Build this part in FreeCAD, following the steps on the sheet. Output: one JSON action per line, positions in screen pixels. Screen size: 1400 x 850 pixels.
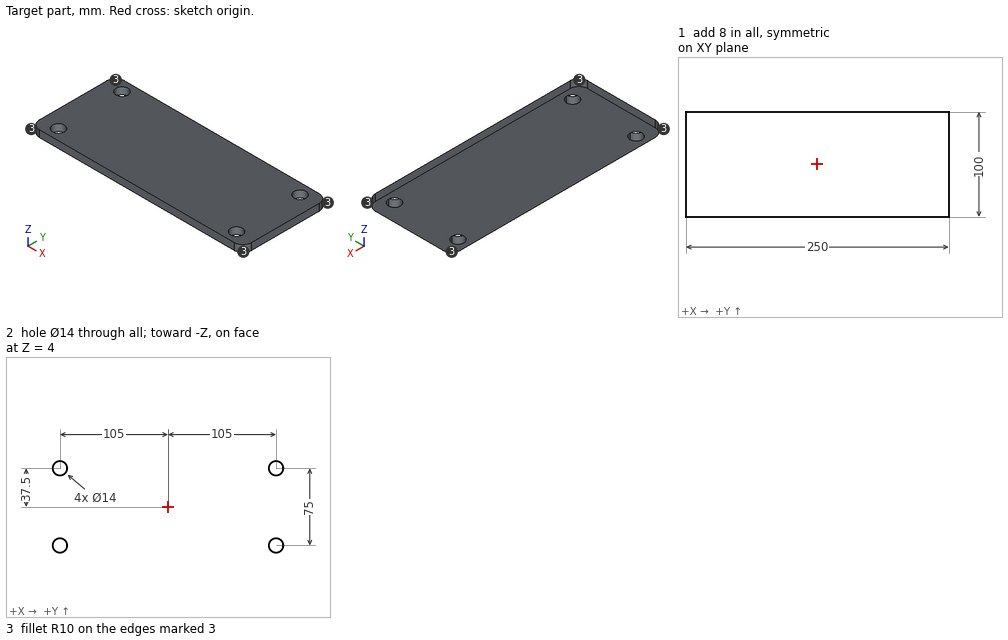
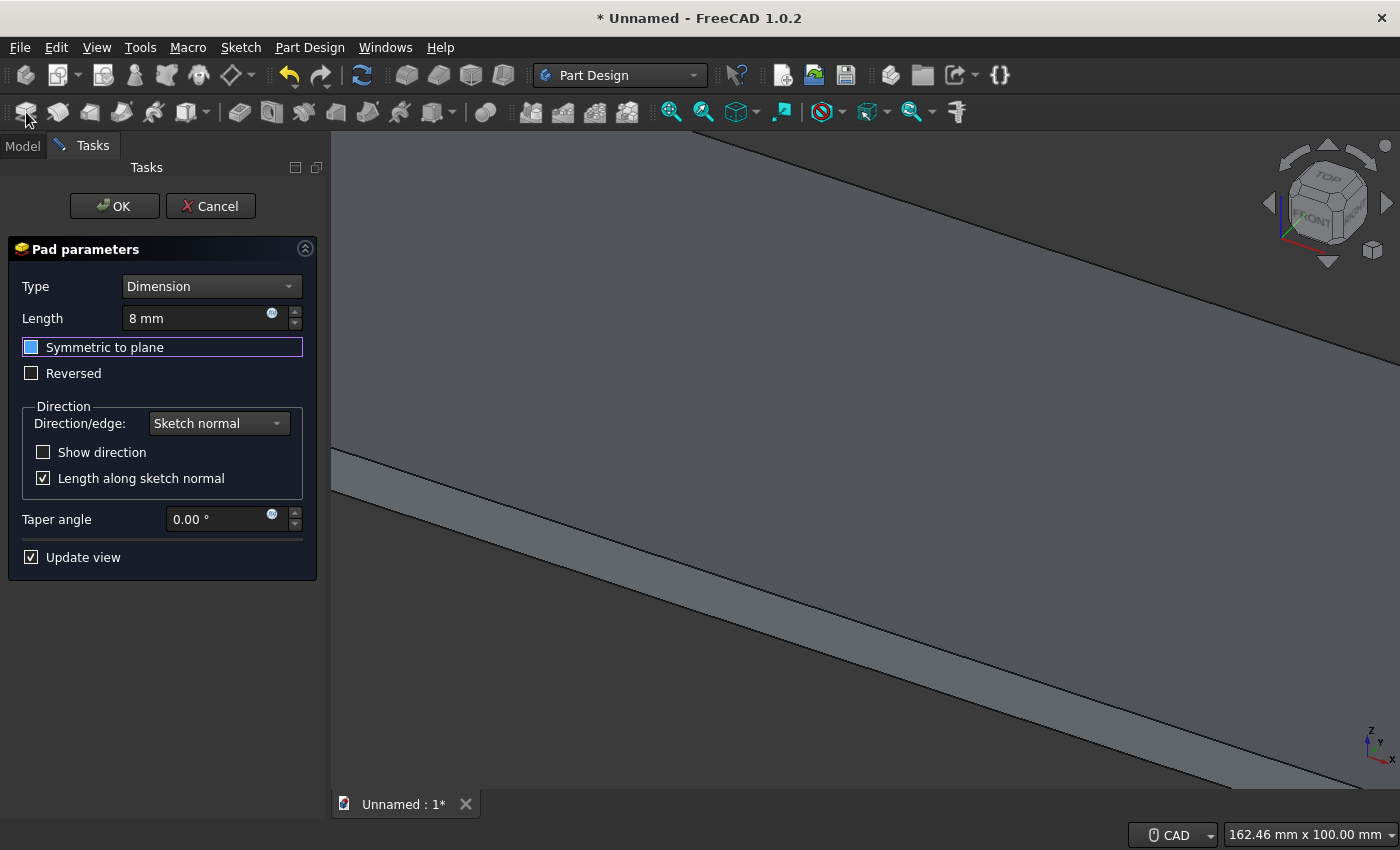
{"action": "left_click", "coordinate": [30, 347]}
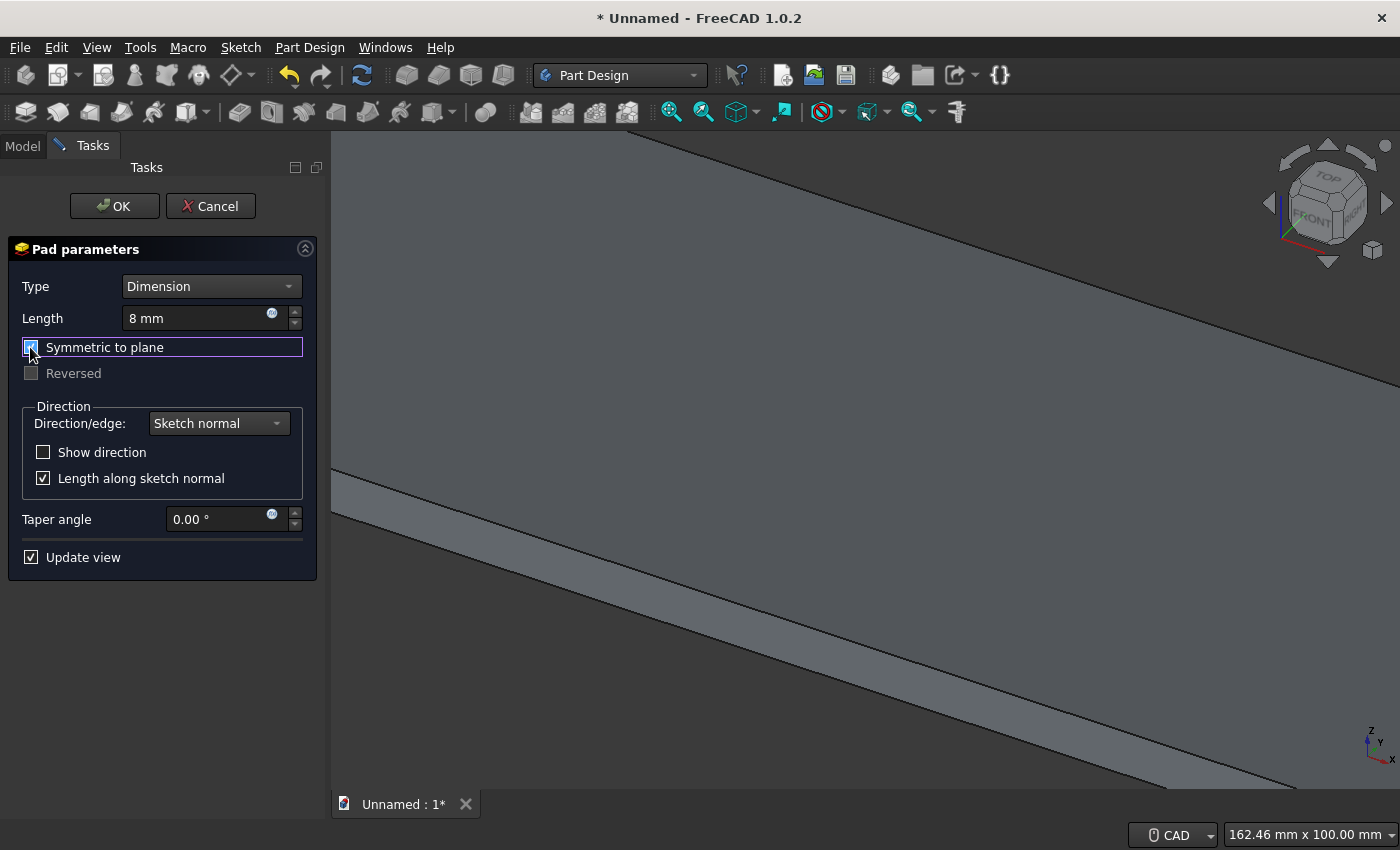
{"action": "left_click", "coordinate": [115, 206]}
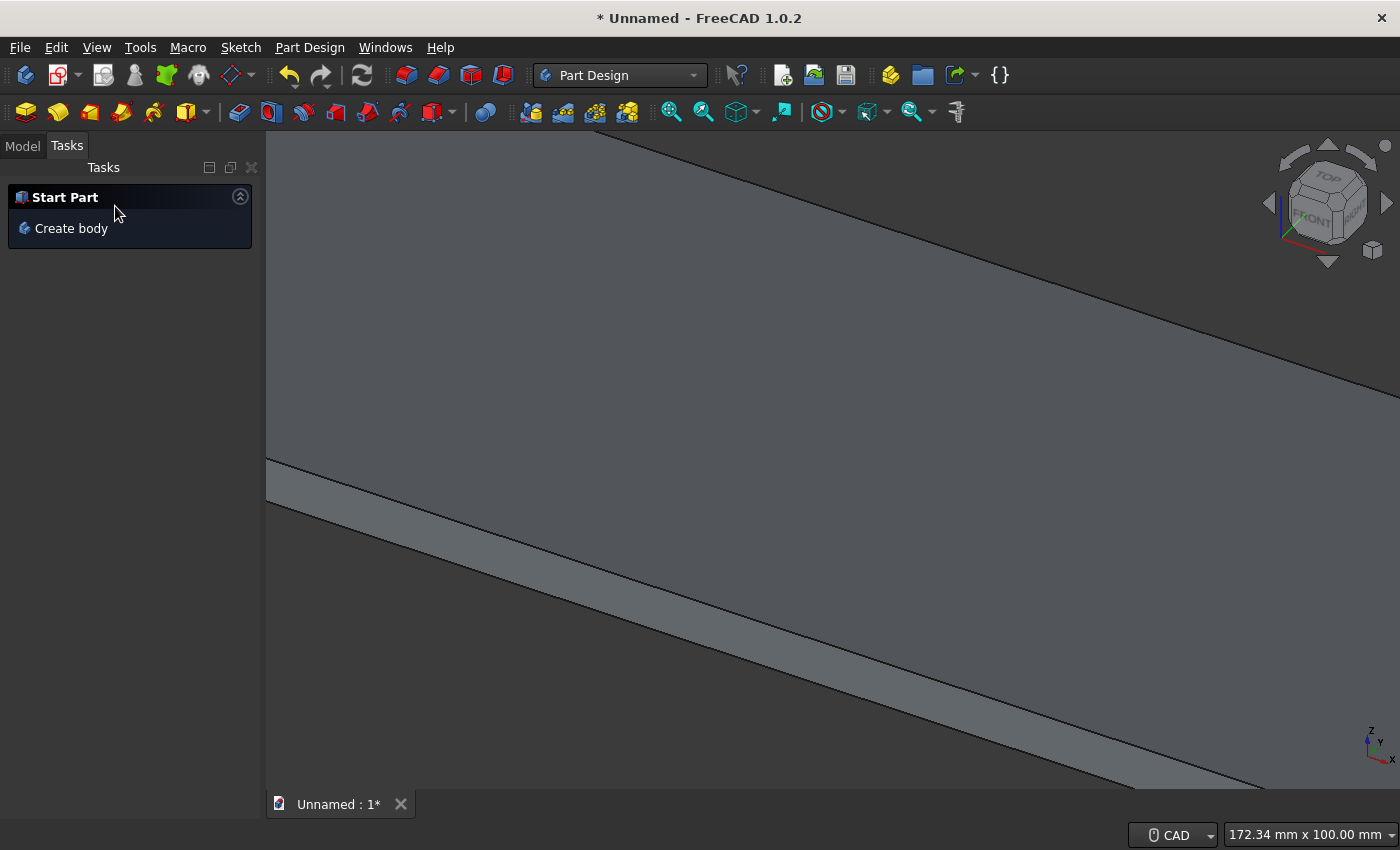
{"action": "left_click", "coordinate": [672, 112]}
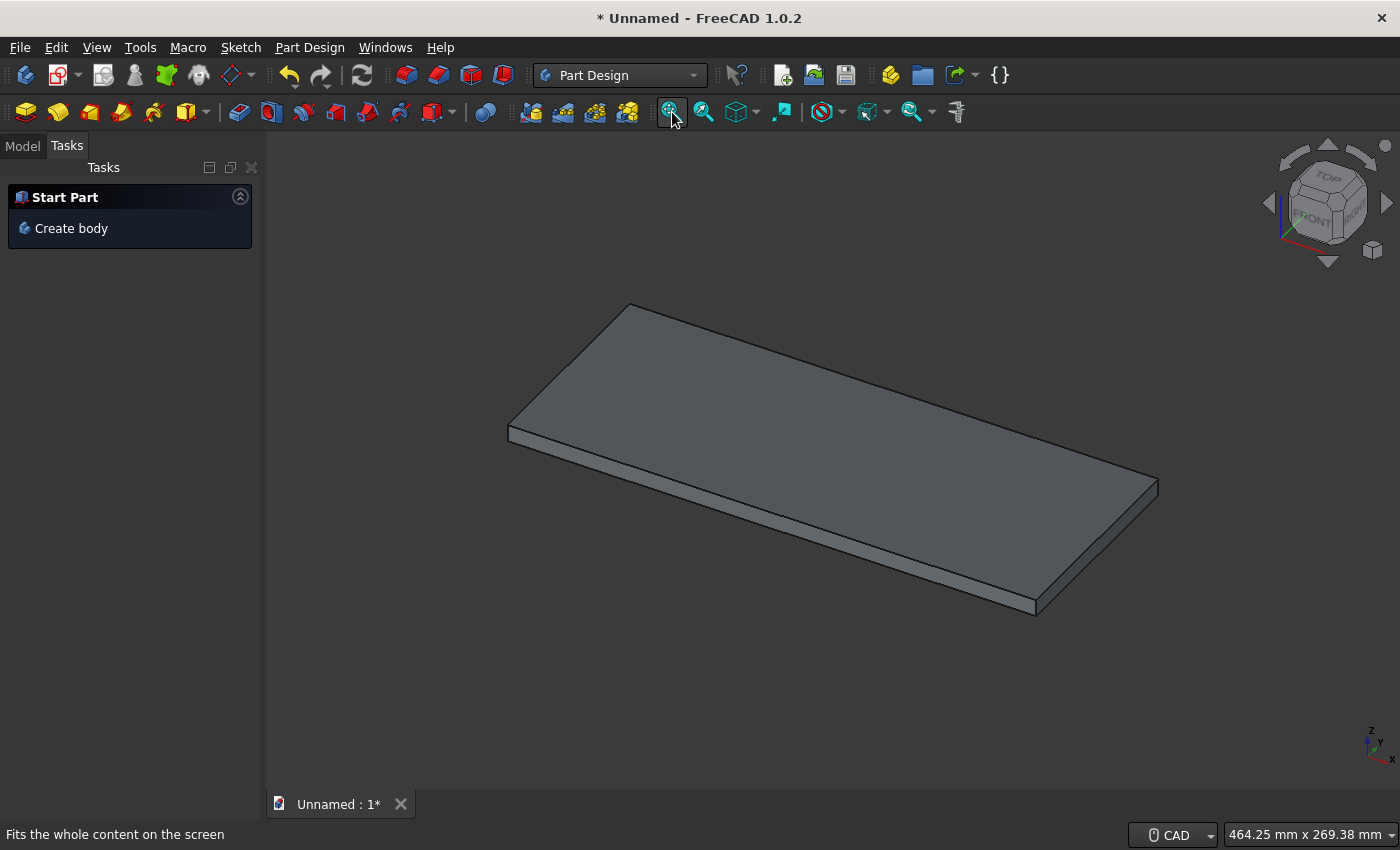
{"action": "left_click", "coordinate": [984, 501]}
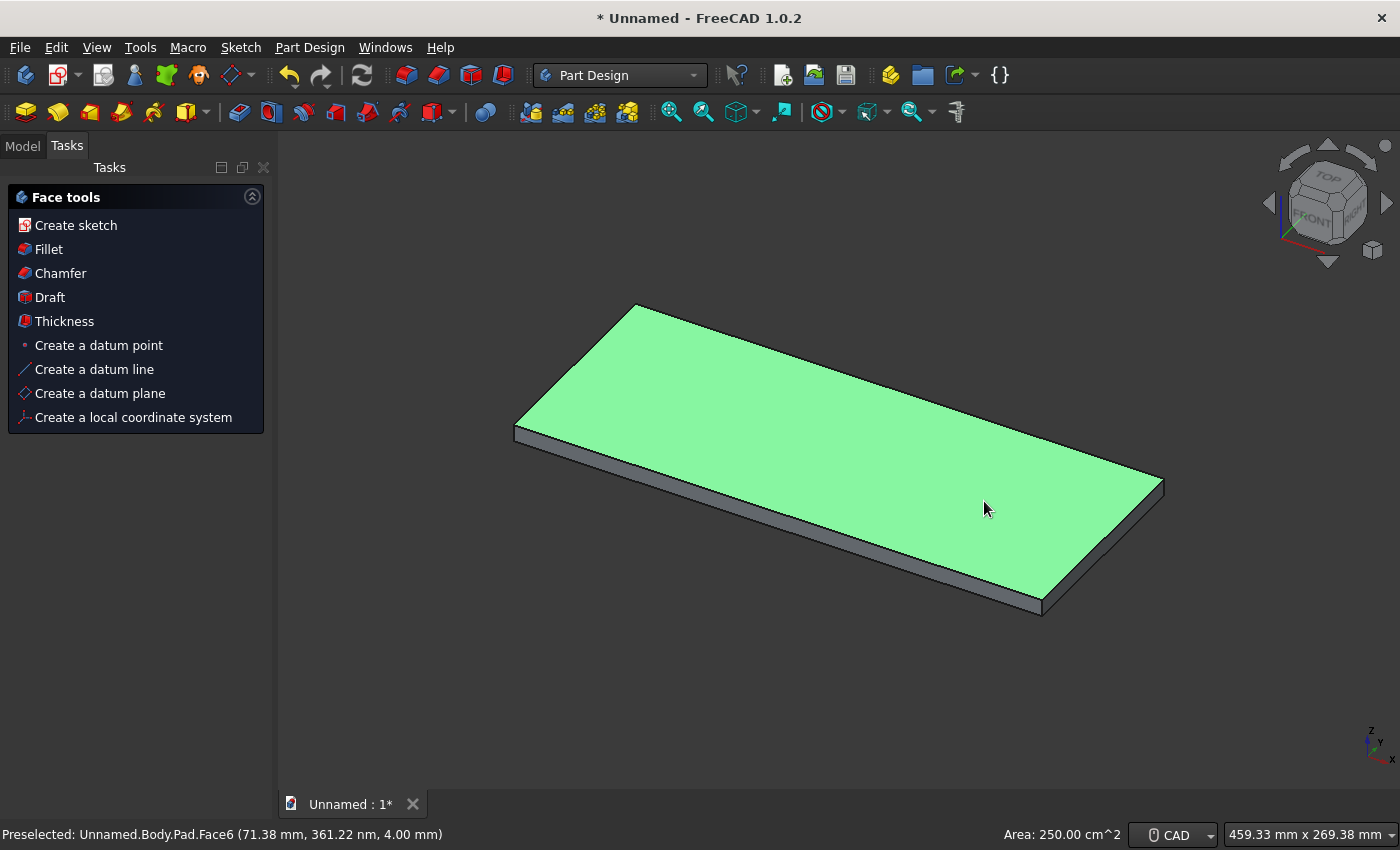
{"action": "left_click", "coordinate": [58, 76]}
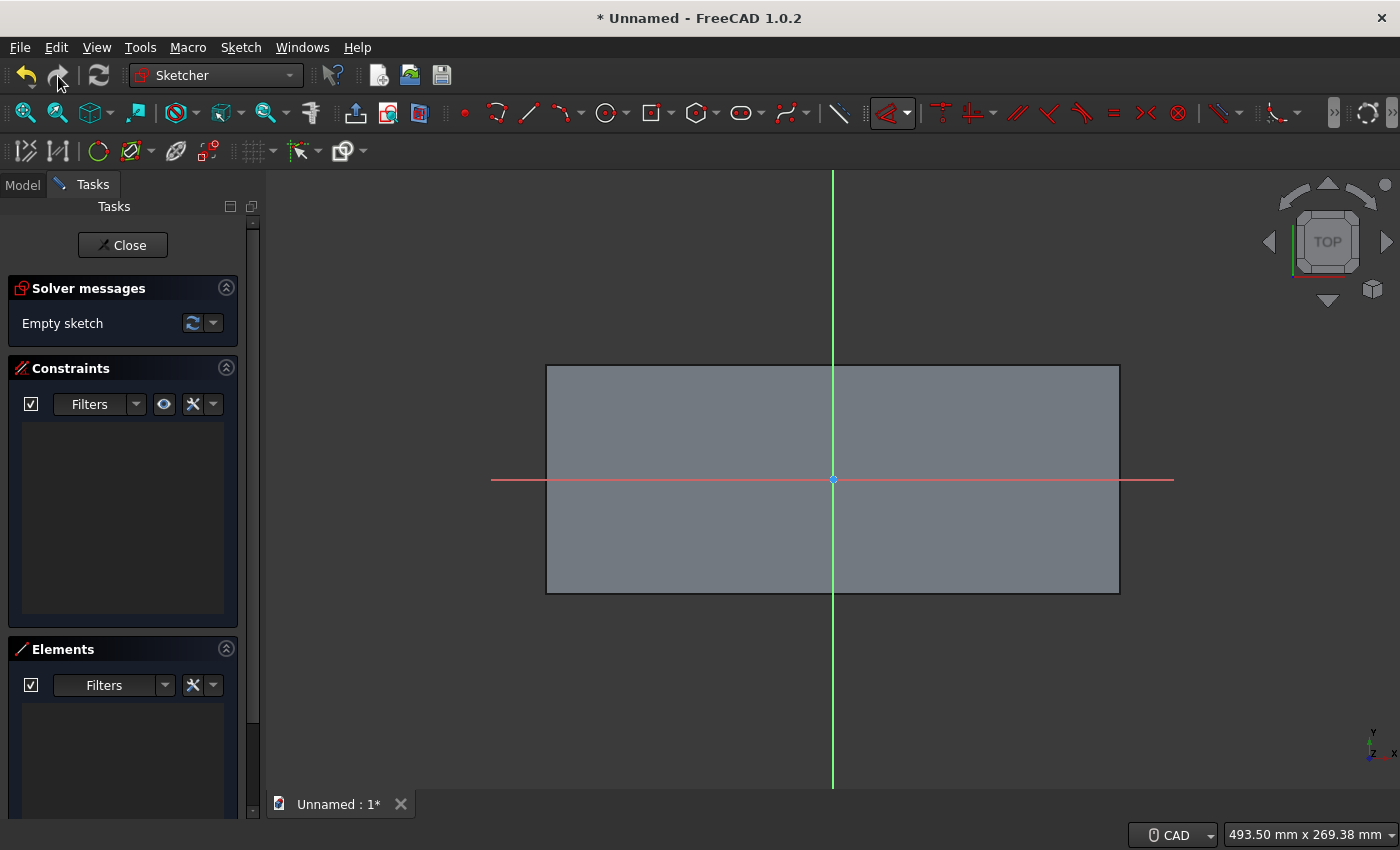
{"action": "left_click", "coordinate": [606, 114]}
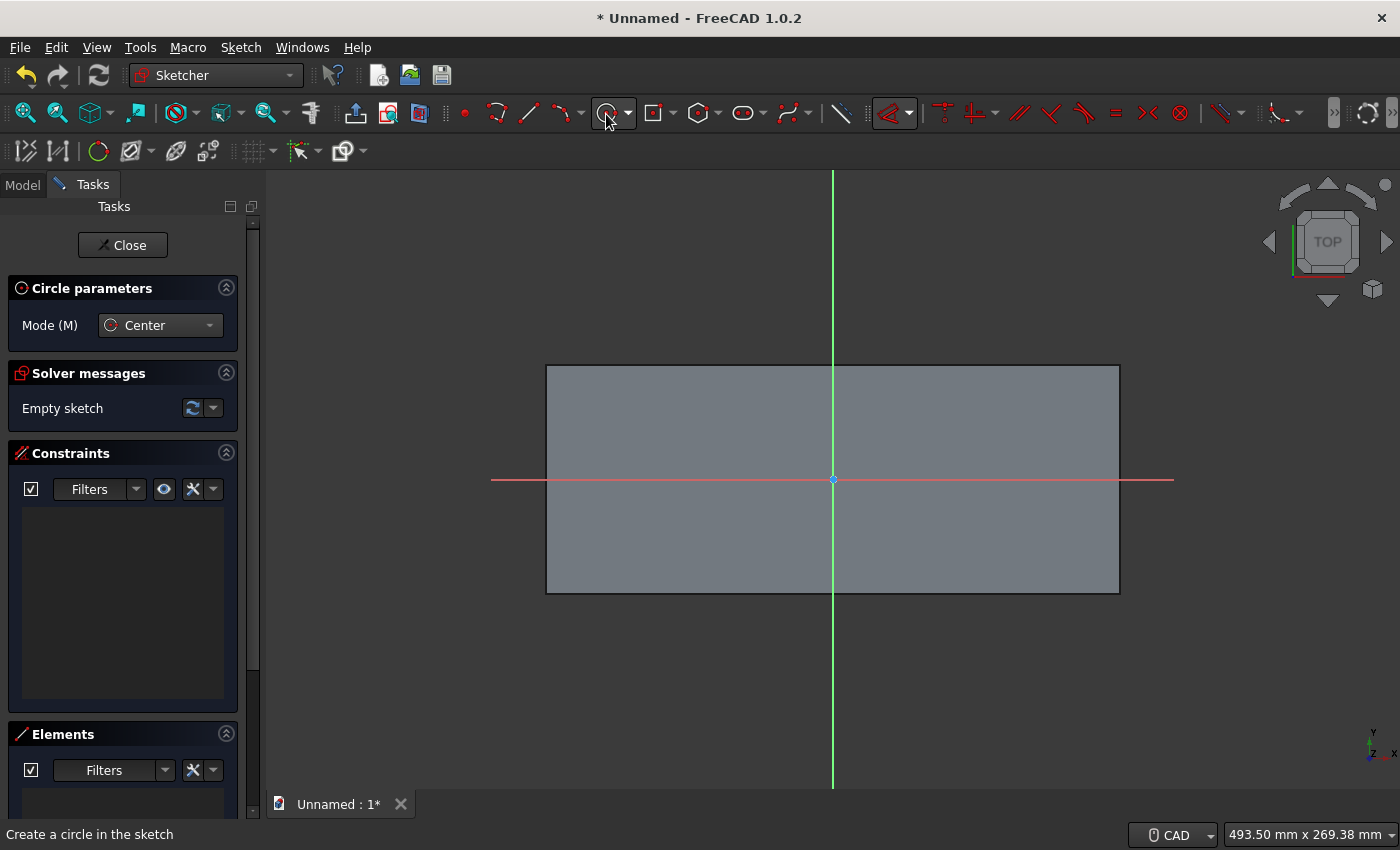
{"action": "scroll", "coordinate": [592, 393], "scroll_direction": "up", "scroll_amount": 2}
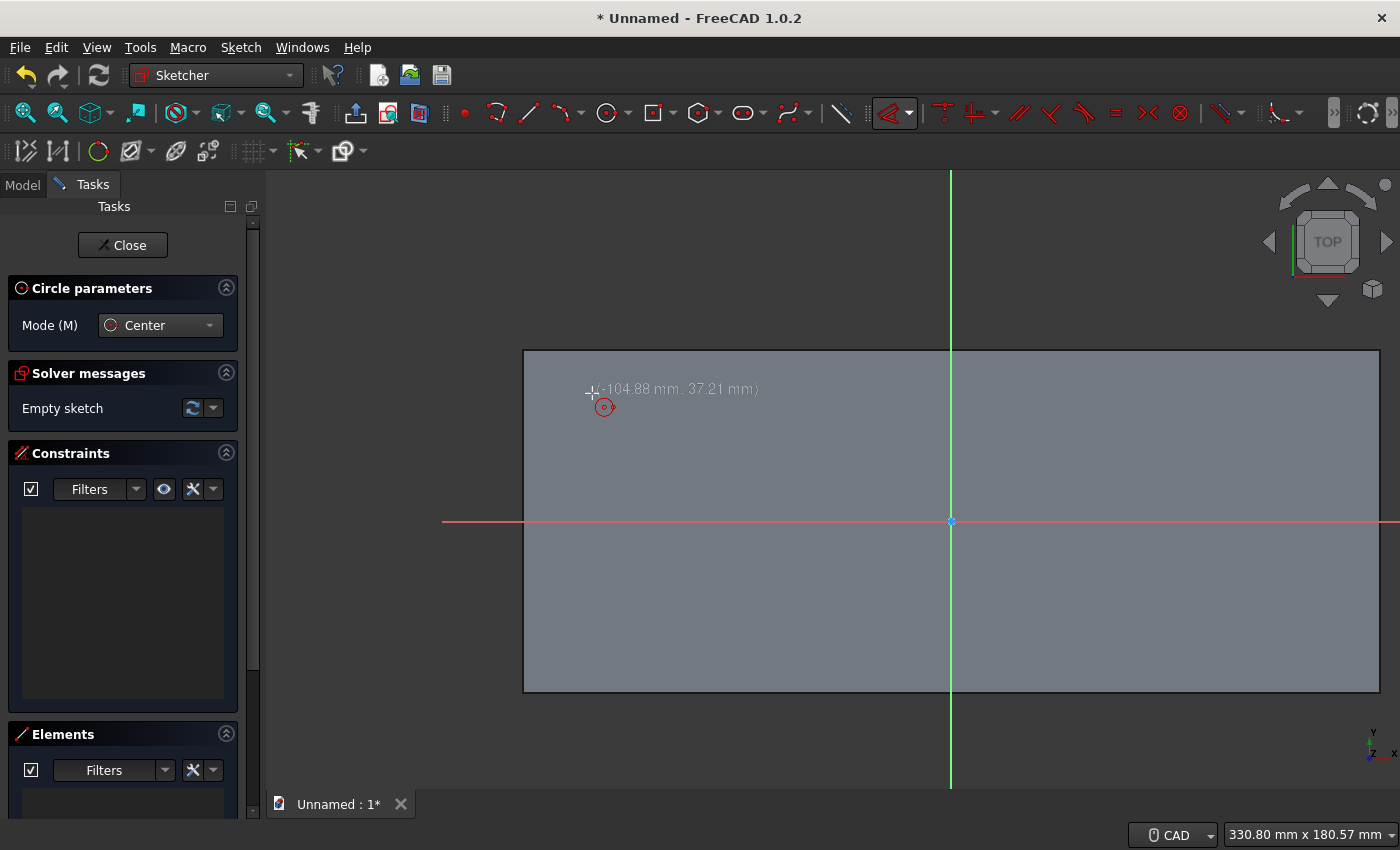
{"action": "left_click", "coordinate": [591, 393]}
{"action": "left_click", "coordinate": [608, 376]}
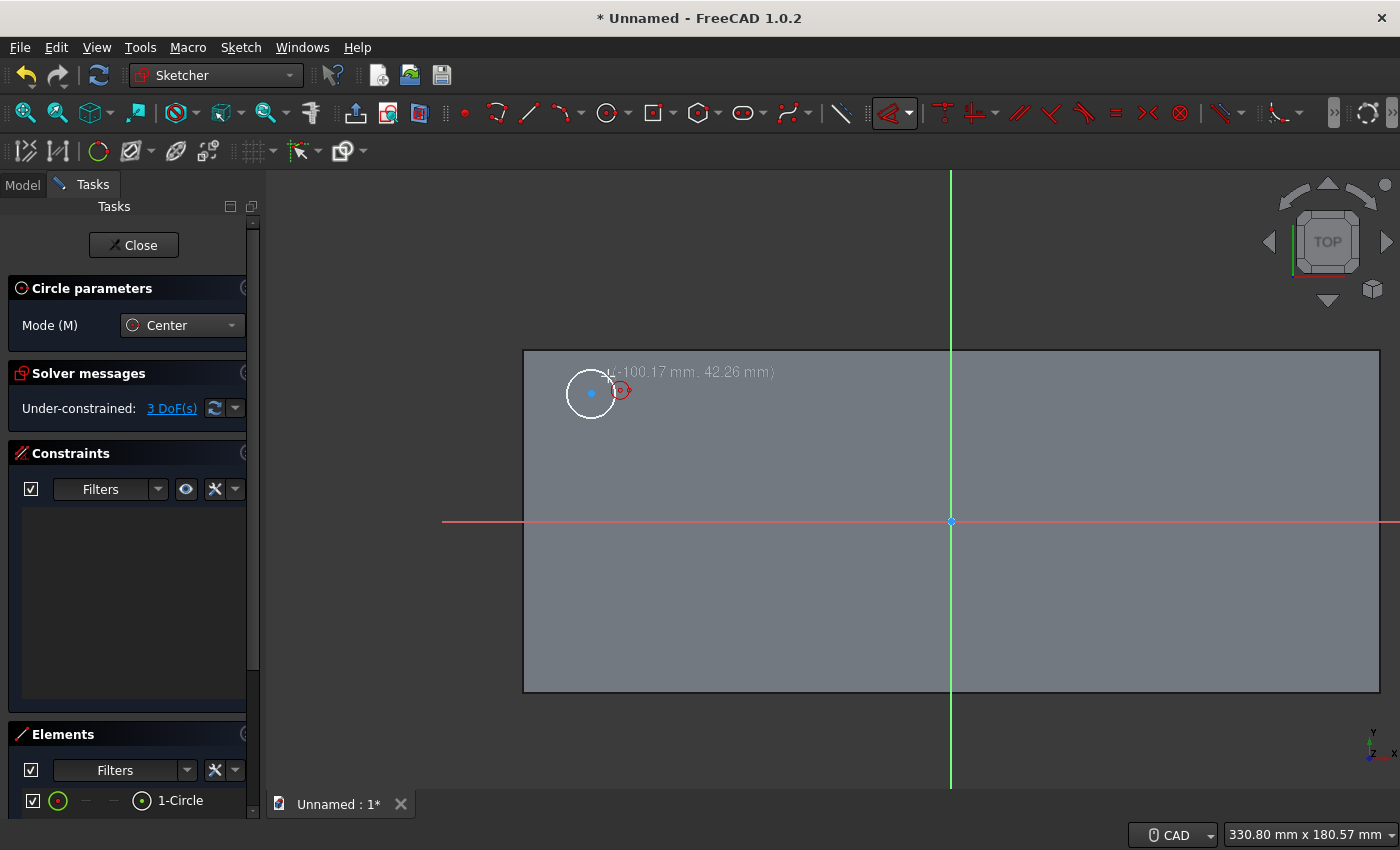
{"action": "scroll", "coordinate": [294, 288], "scroll_direction": "down", "scroll_amount": 1}